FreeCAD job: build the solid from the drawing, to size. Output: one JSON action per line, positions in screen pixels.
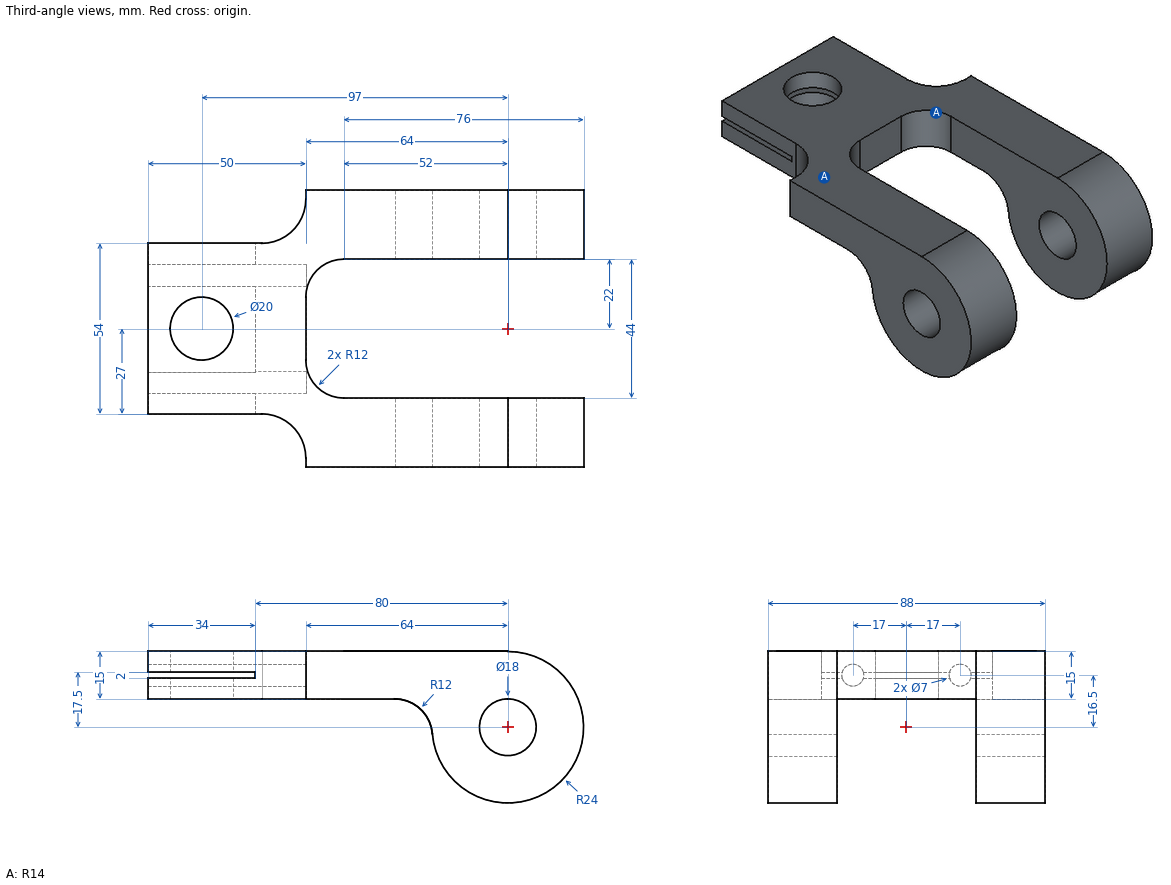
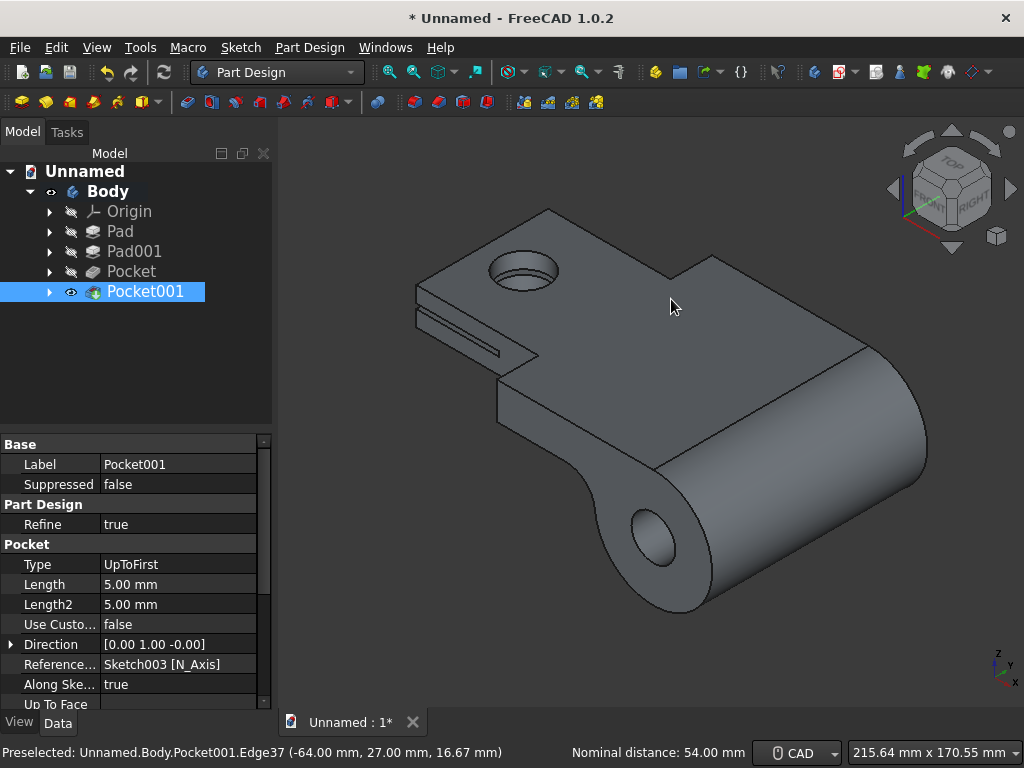
{"action": "left_click", "coordinate": [416, 102]}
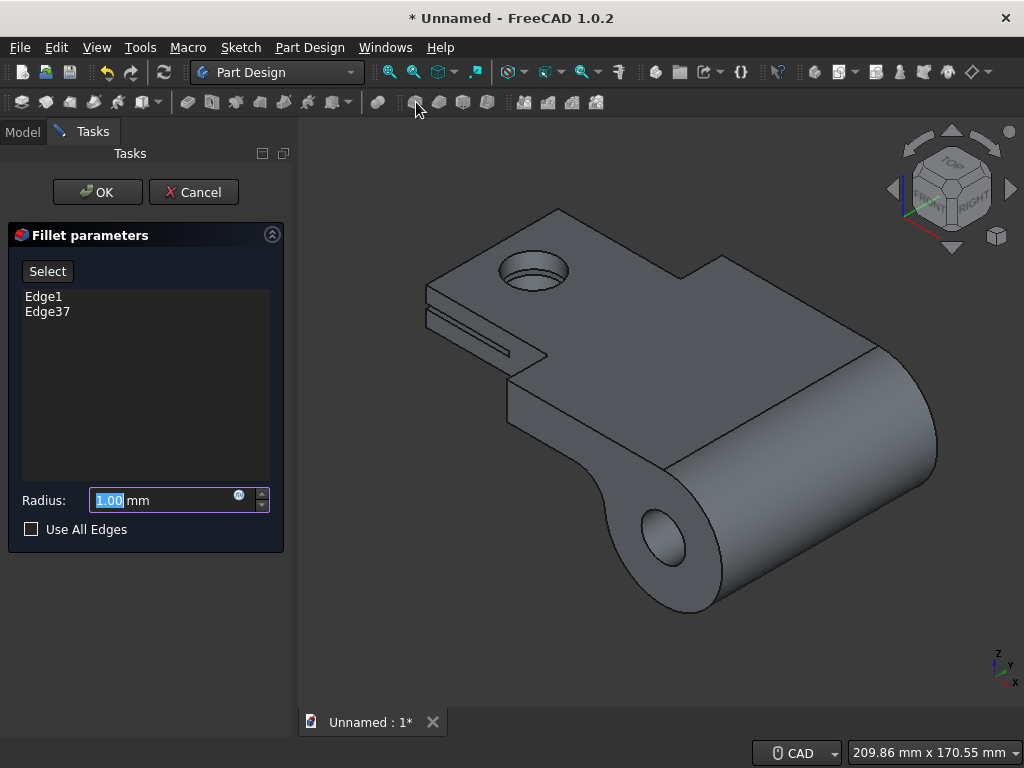
{"action": "type", "text": "14"}
{"action": "key", "text": "Tab"}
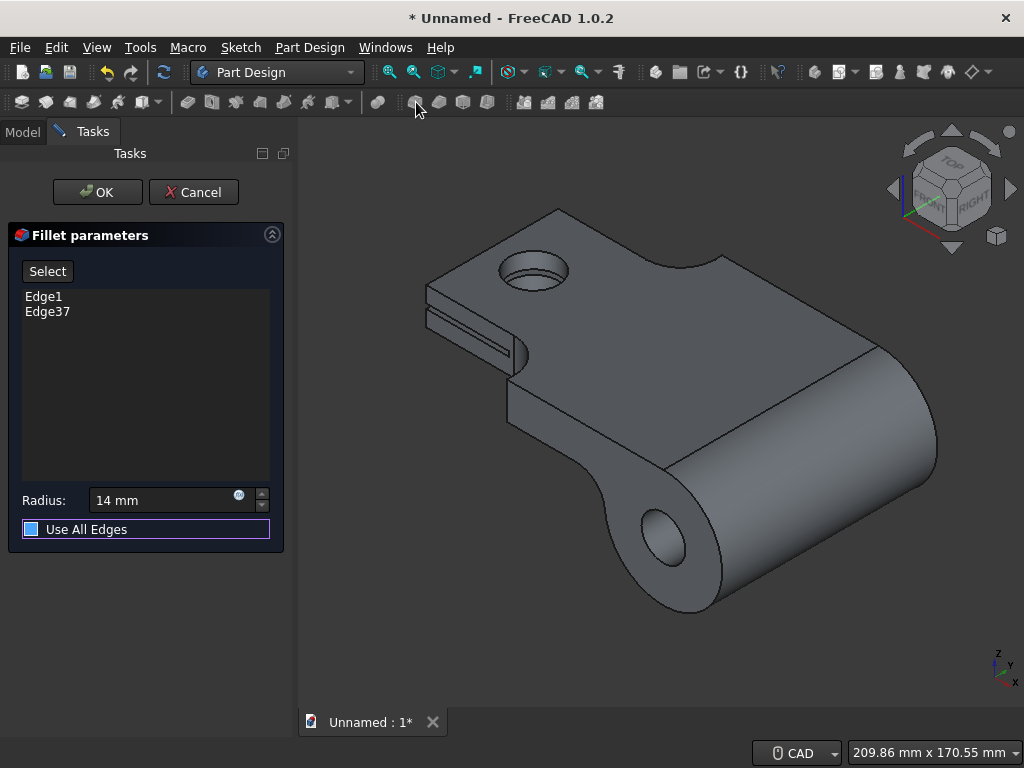
{"action": "left_click", "coordinate": [98, 192]}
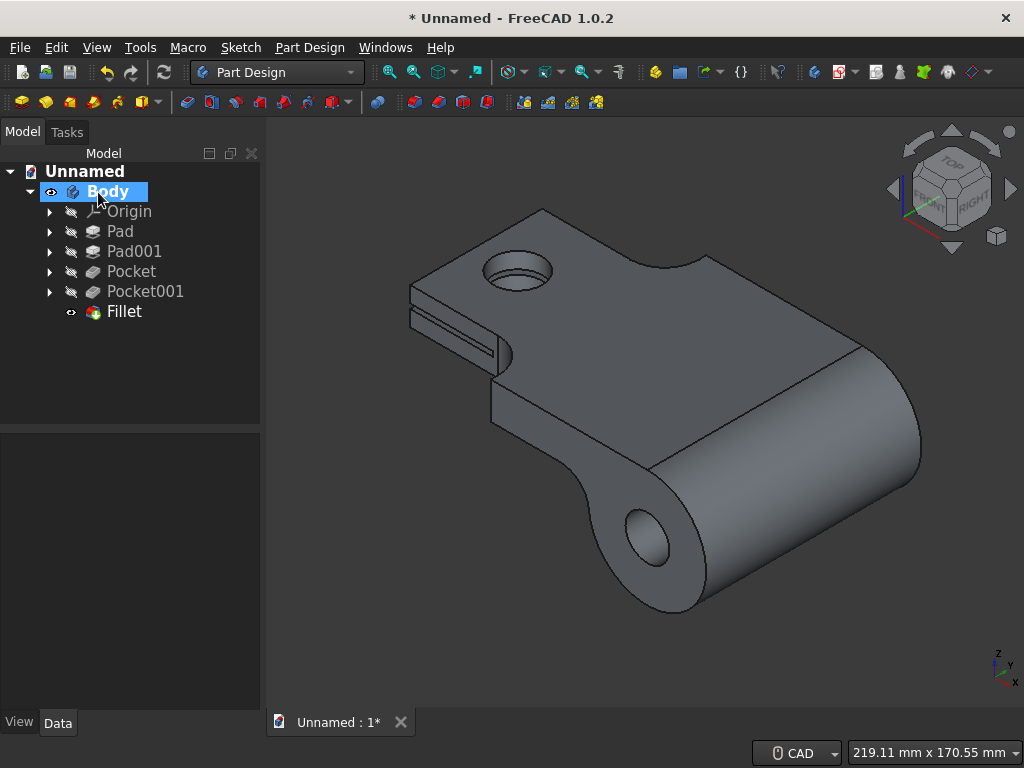
{"action": "key", "text": "6"}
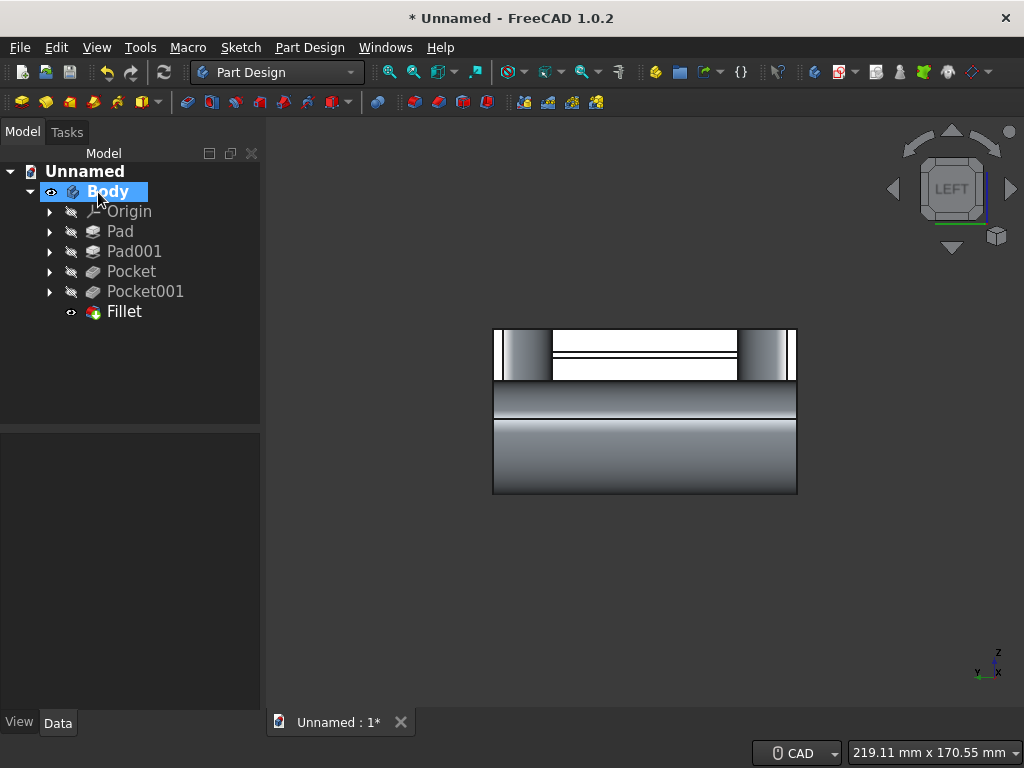
{"action": "left_click", "coordinate": [390, 72]}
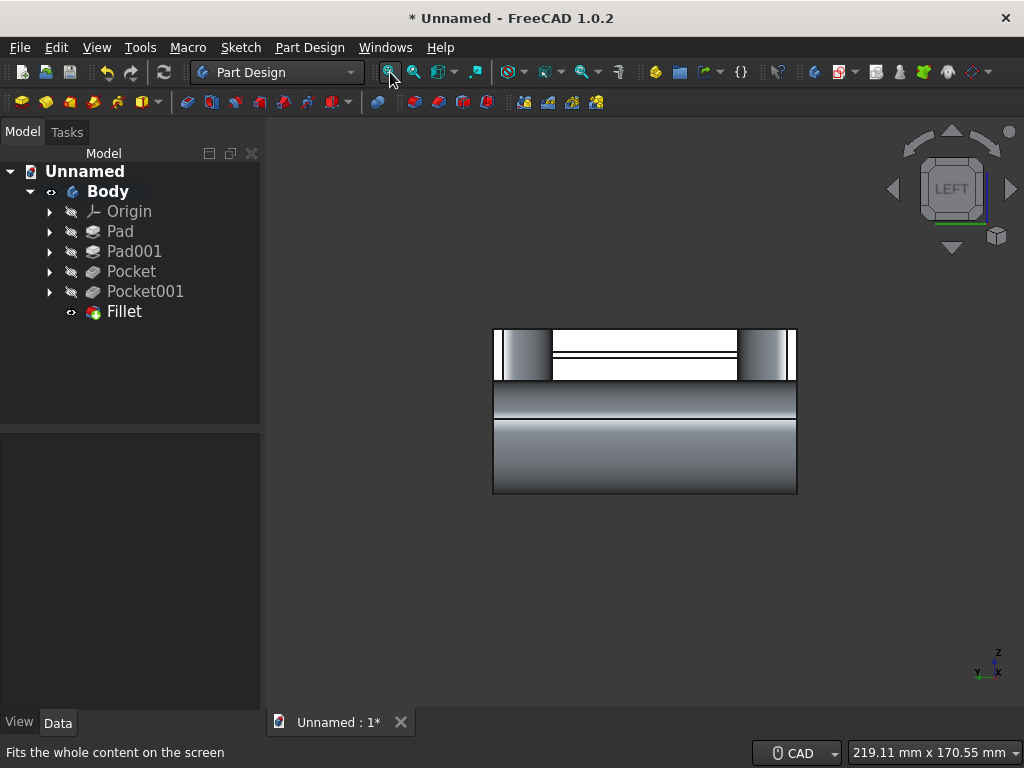
{"action": "left_click", "coordinate": [565, 339]}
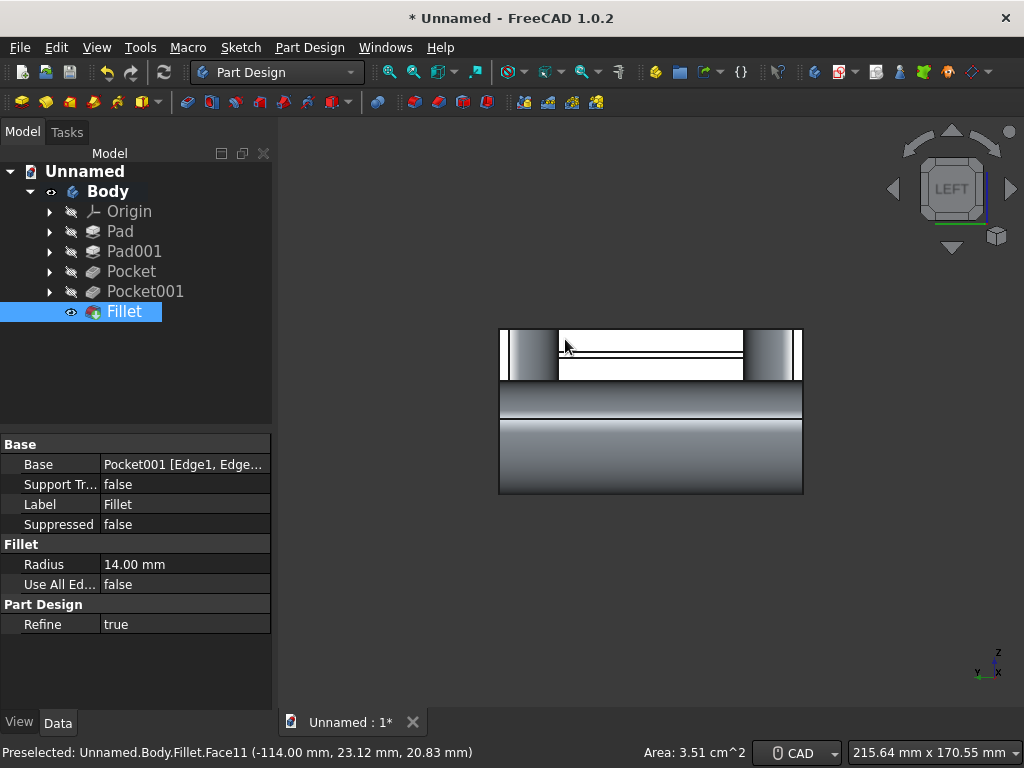
{"action": "left_click", "coordinate": [840, 72]}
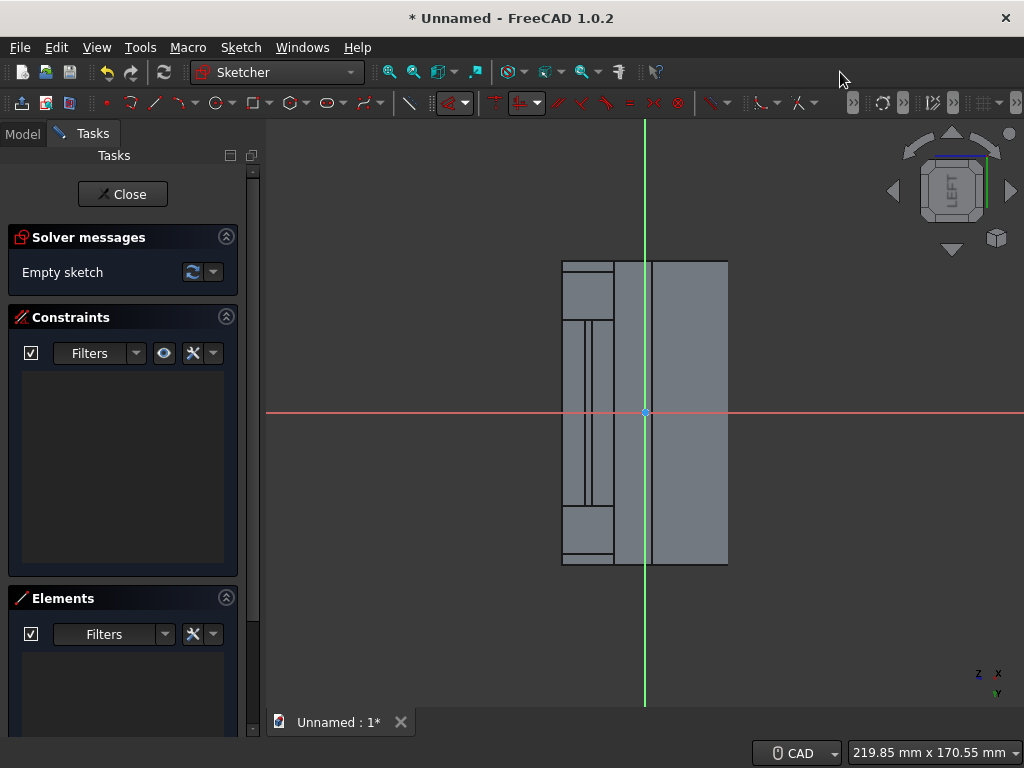
{"action": "scroll", "coordinate": [630, 413], "scroll_direction": "up", "scroll_amount": 5}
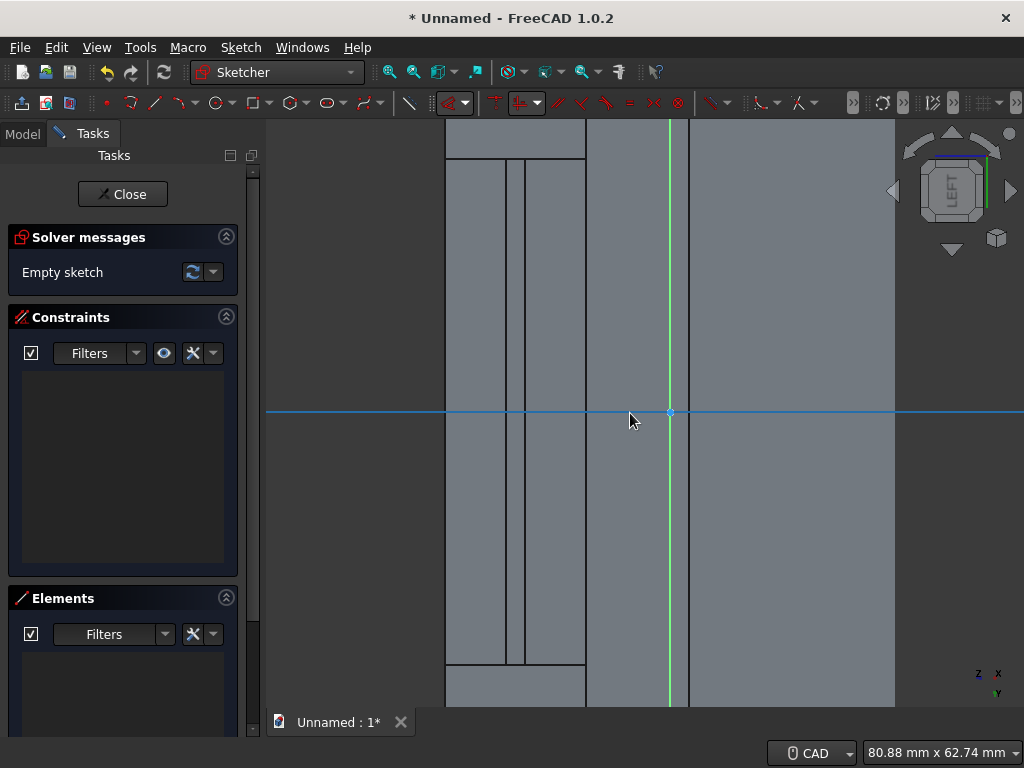
{"action": "left_click", "coordinate": [216, 104]}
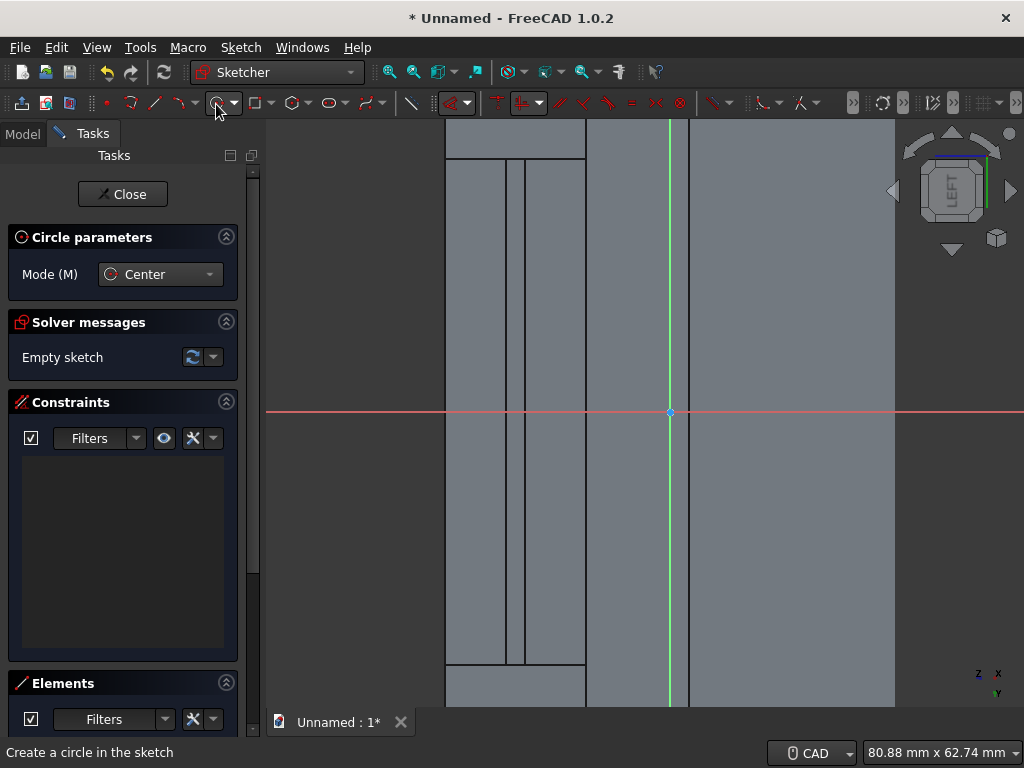
{"action": "left_click", "coordinate": [515, 571]}
{"action": "left_click", "coordinate": [539, 548]}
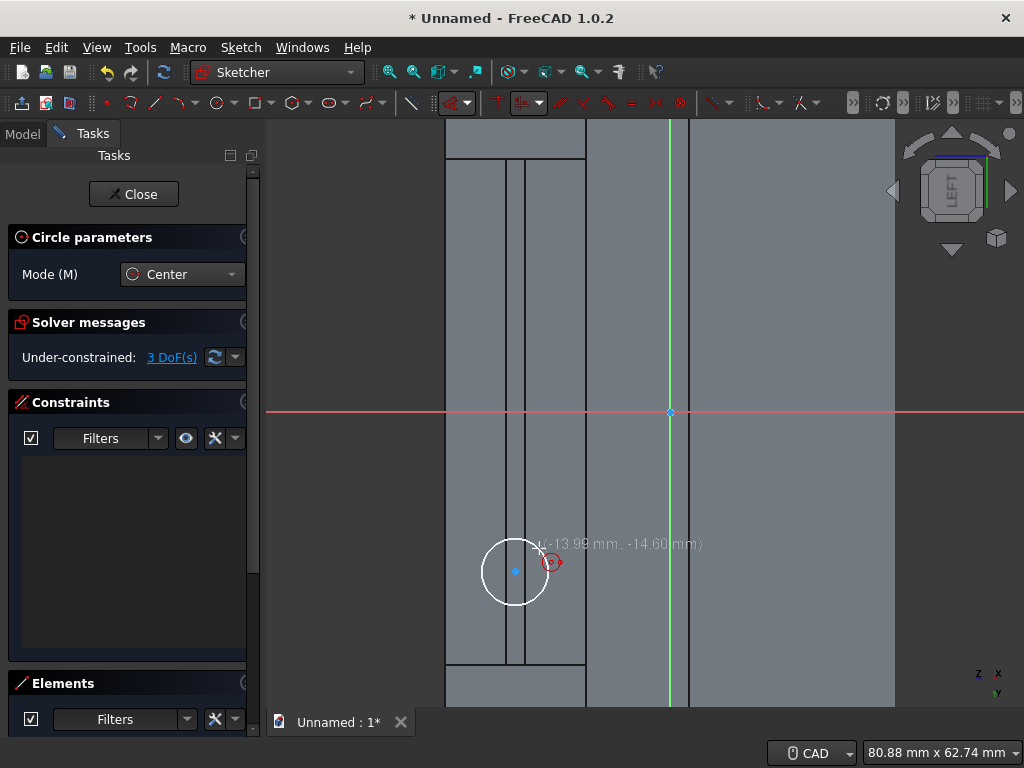
{"action": "left_click", "coordinate": [515, 253]}
{"action": "left_click", "coordinate": [539, 230]}
{"action": "key", "text": "Escape"}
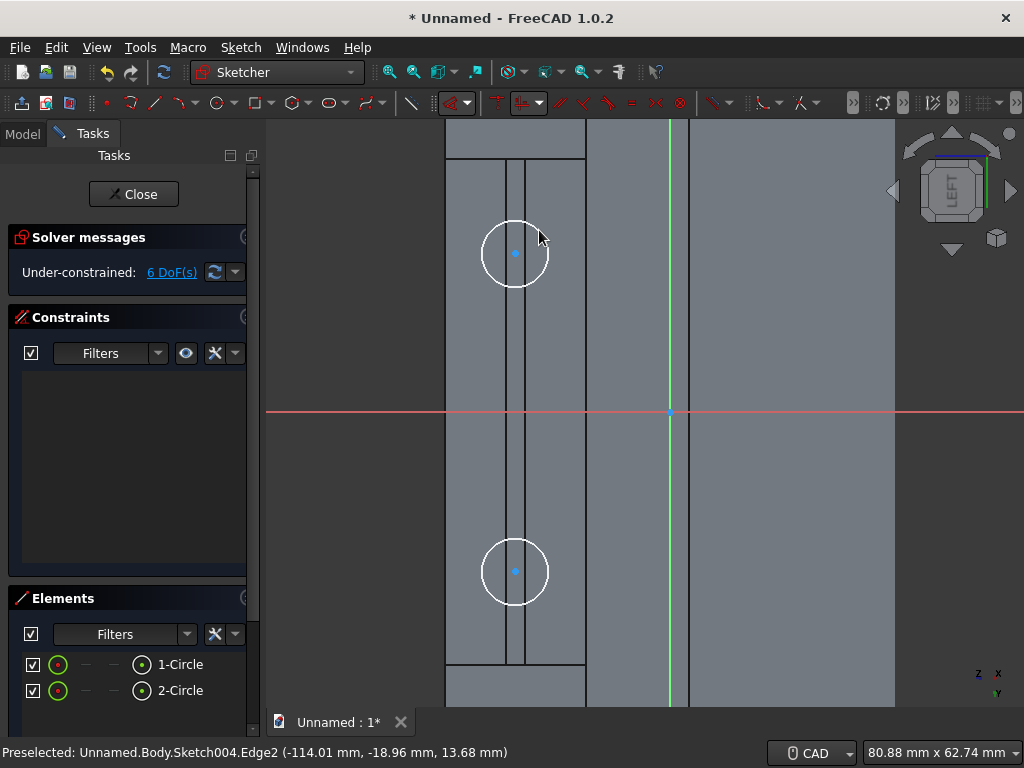
{"action": "left_click", "coordinate": [538, 548]}